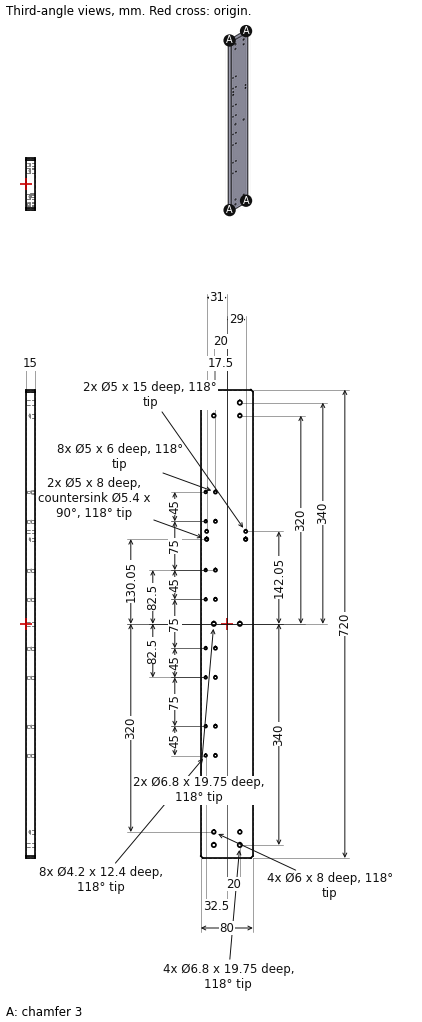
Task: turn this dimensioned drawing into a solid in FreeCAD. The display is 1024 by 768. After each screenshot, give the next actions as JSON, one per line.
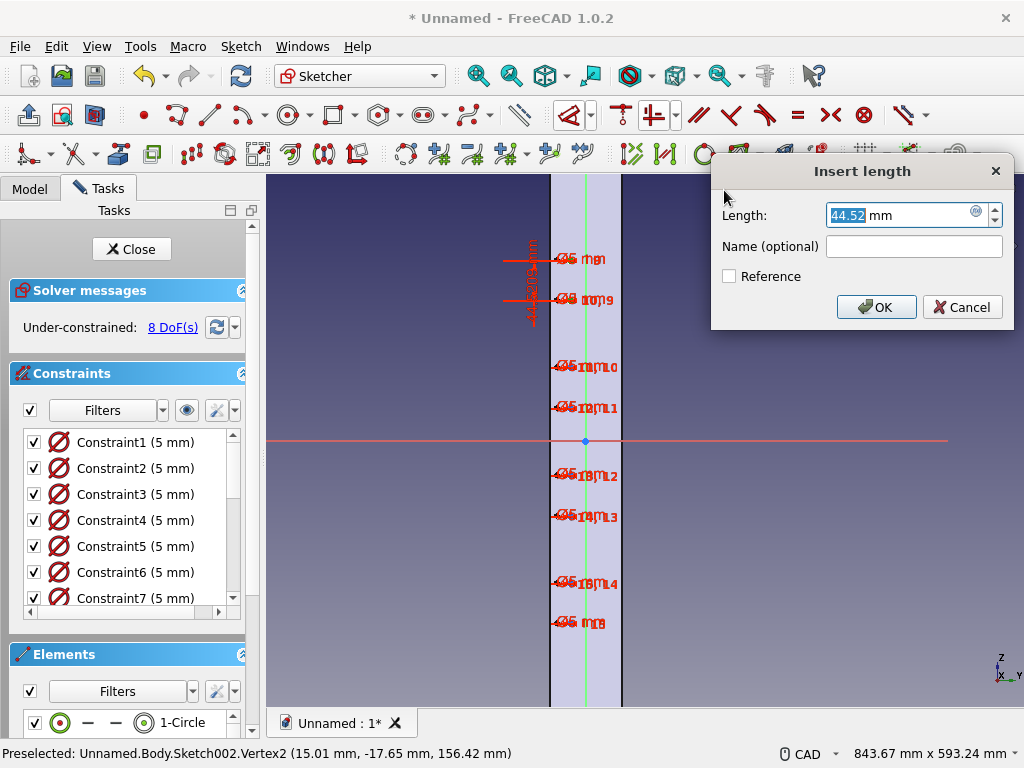
{"action": "type", "text": "45"}
{"action": "key", "text": "Return"}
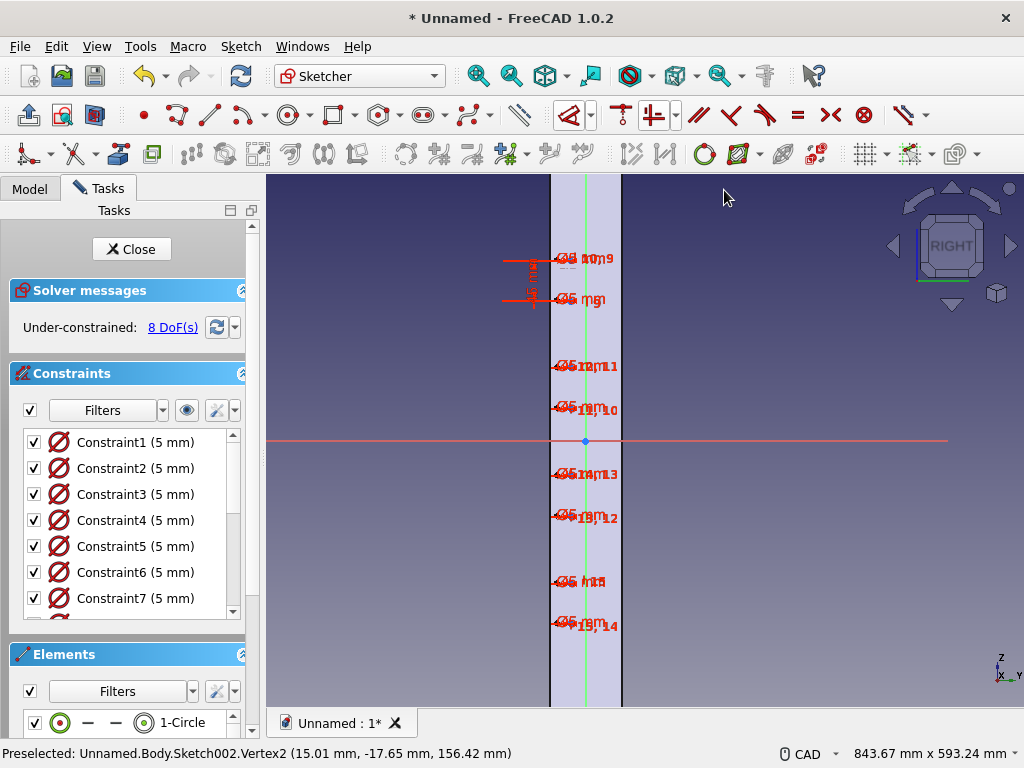
{"action": "left_click", "coordinate": [570, 301]}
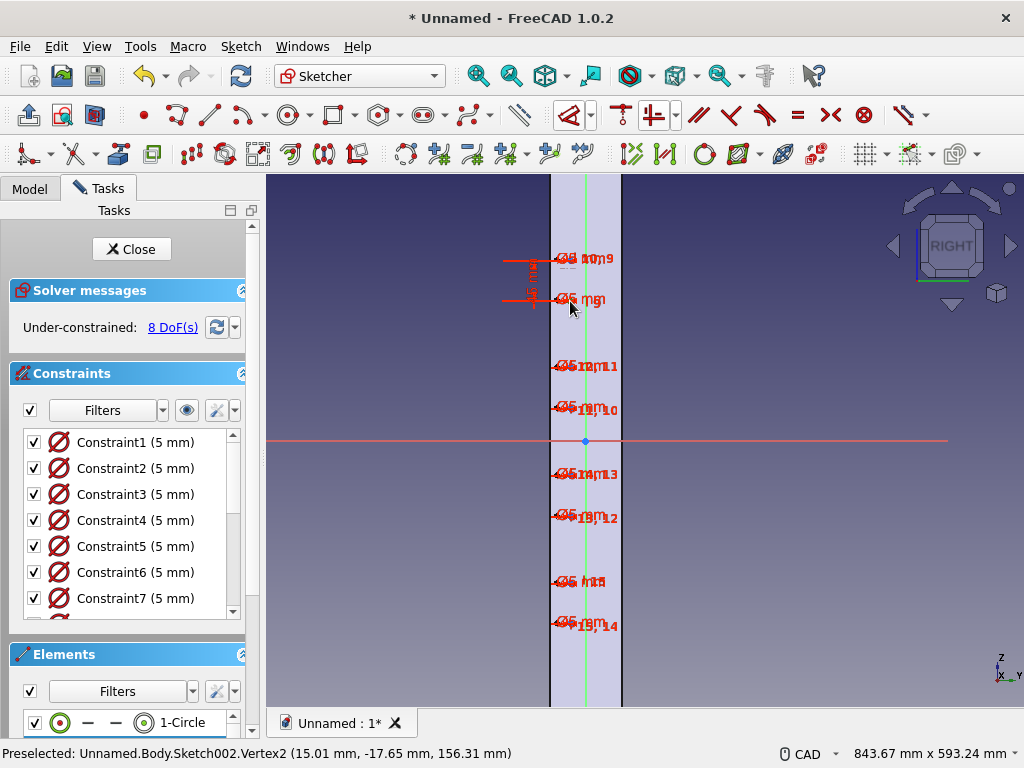
{"action": "left_click", "coordinate": [570, 368]}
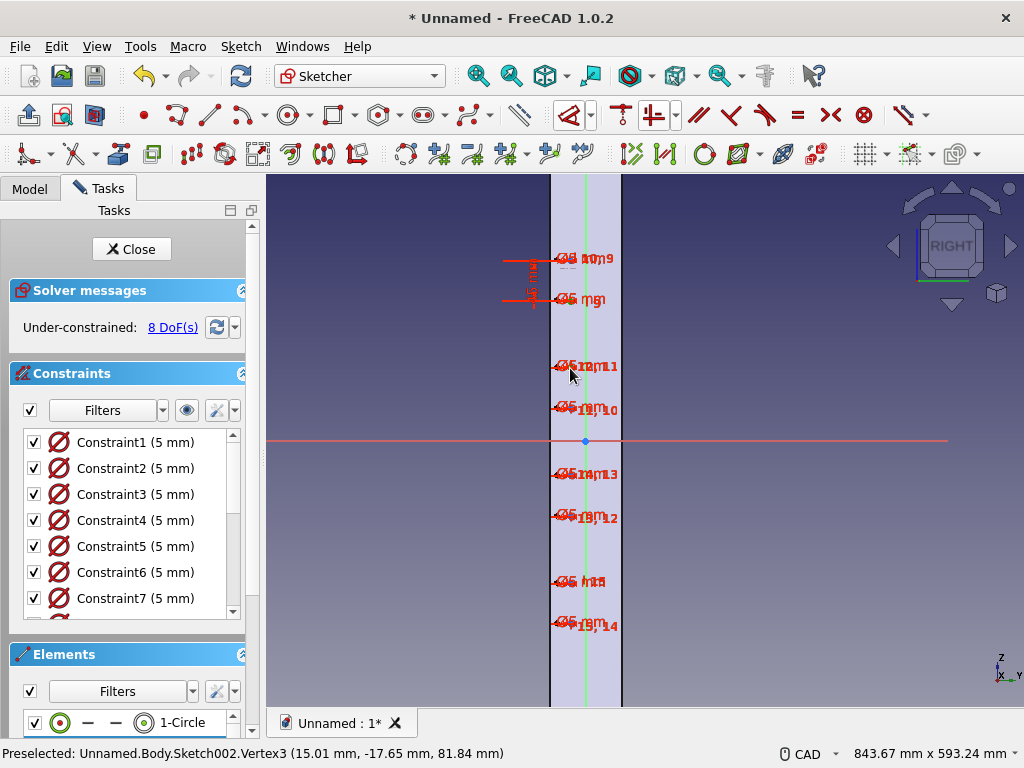
{"action": "left_click", "coordinate": [590, 116]}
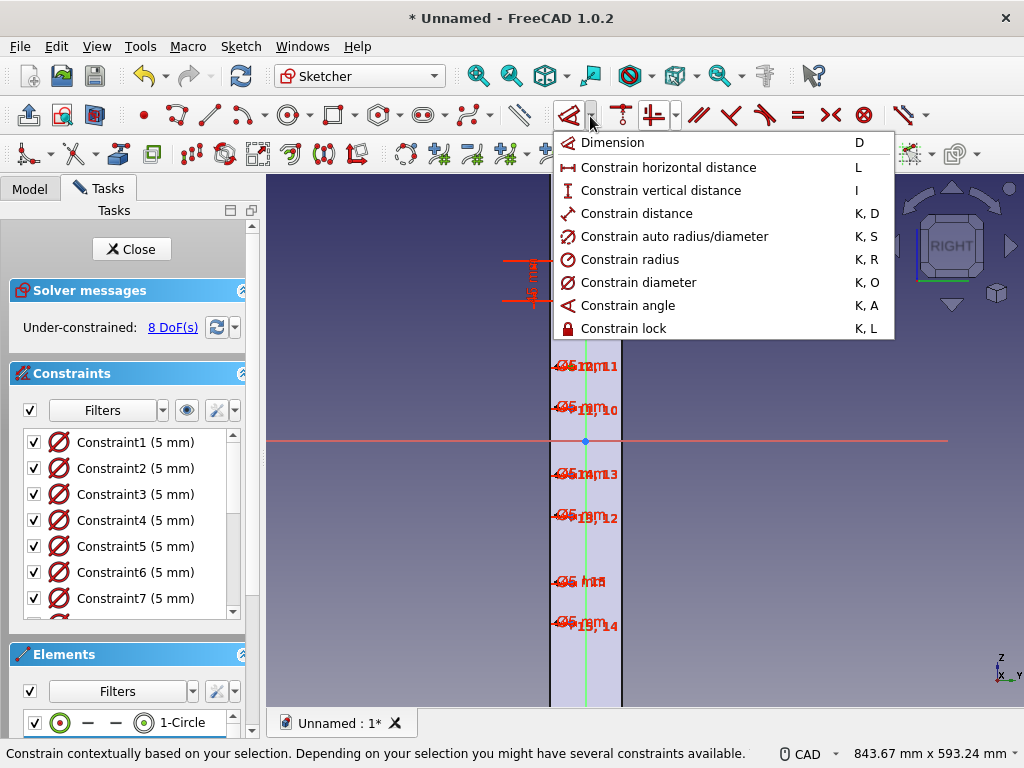
{"action": "left_click", "coordinate": [724, 190]}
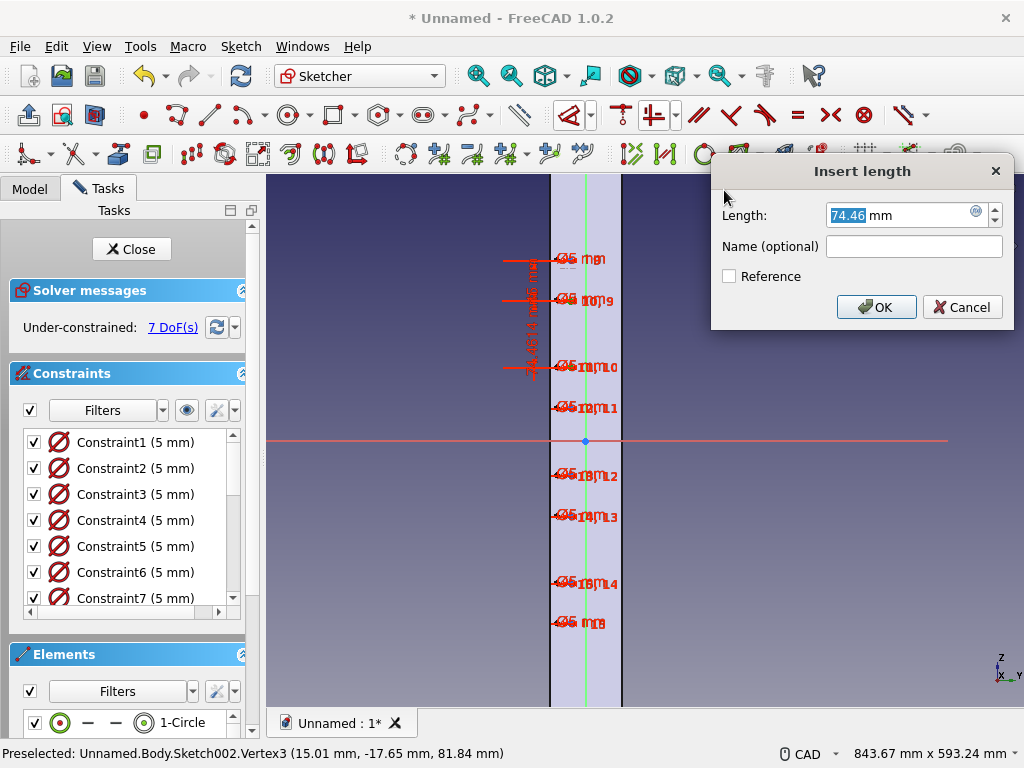
{"action": "type", "text": "75"}
{"action": "key", "text": "Return"}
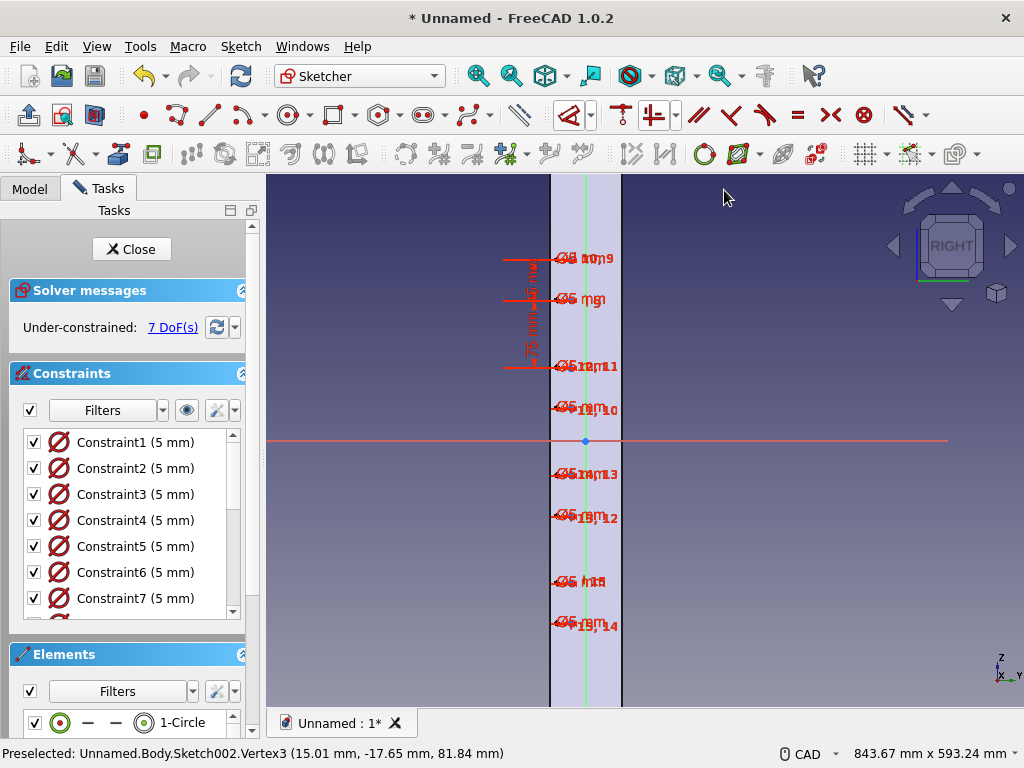
{"action": "left_click", "coordinate": [570, 368]}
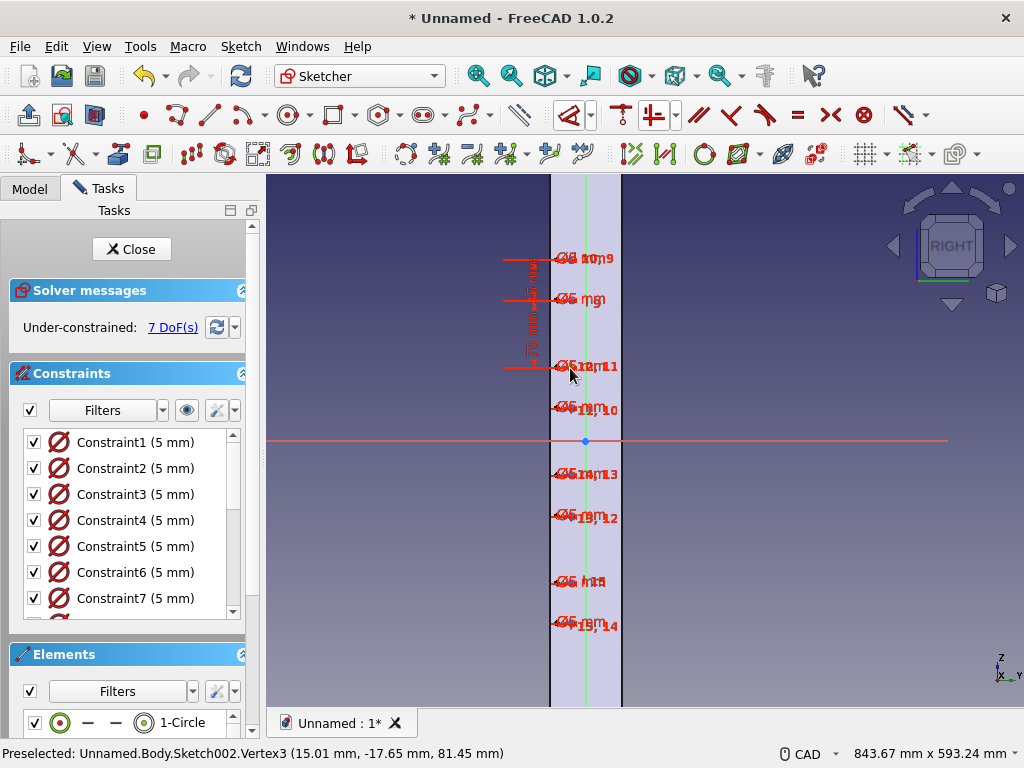
{"action": "left_click", "coordinate": [570, 409]}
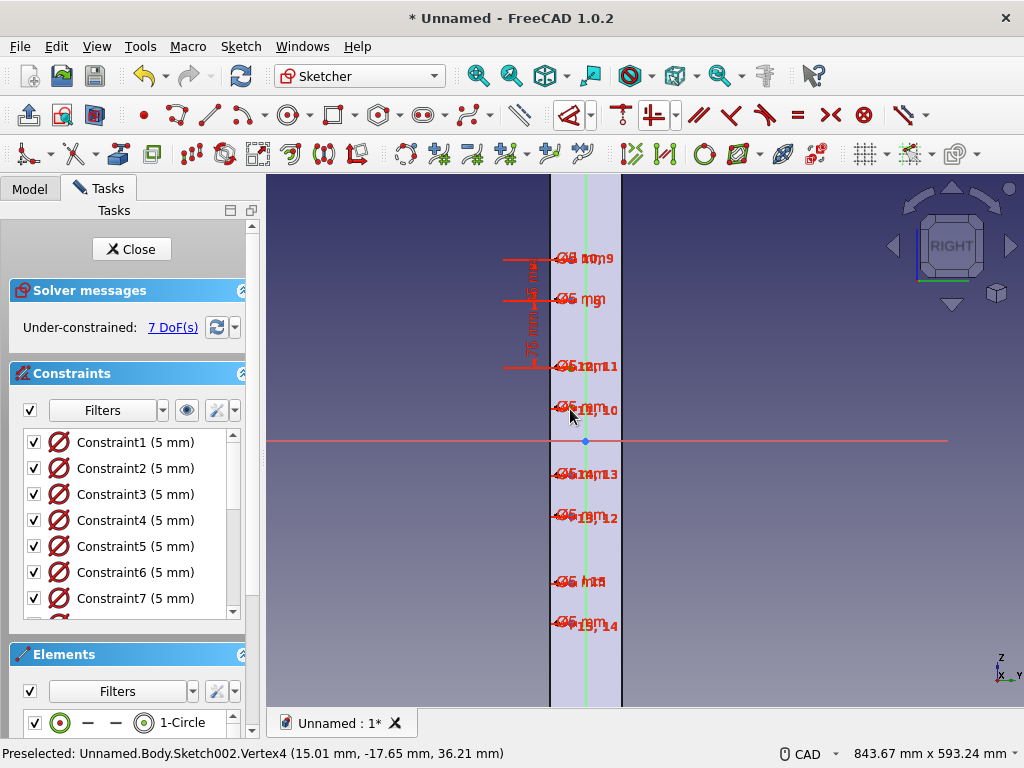
{"action": "left_click", "coordinate": [590, 116]}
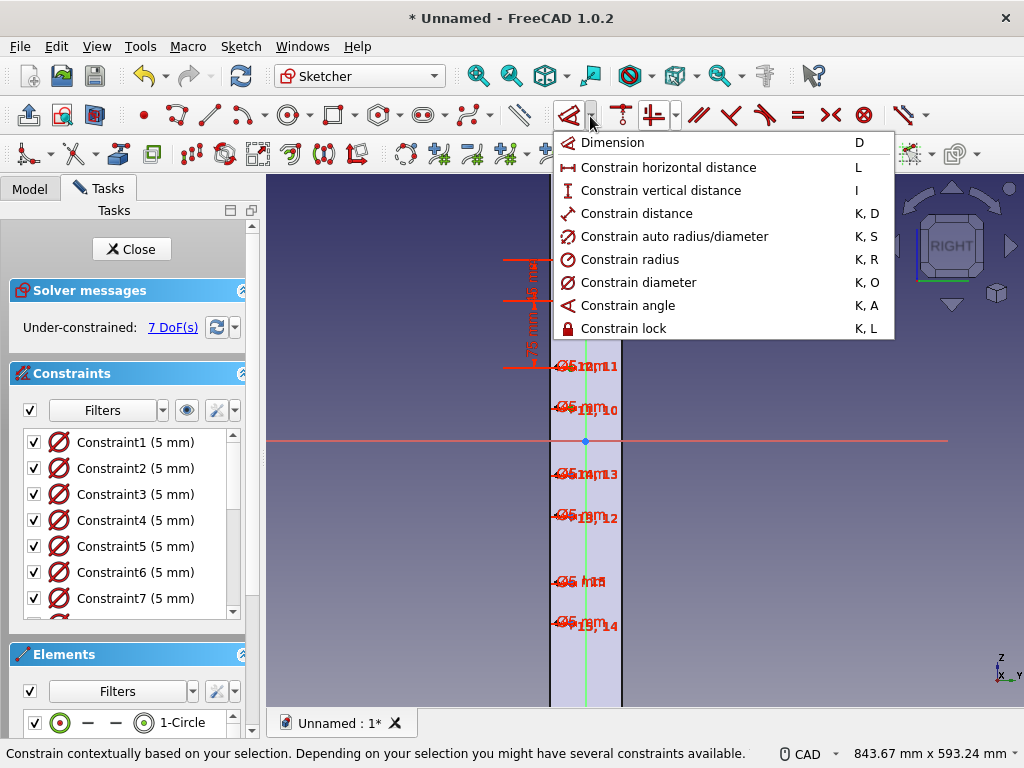
{"action": "left_click", "coordinate": [724, 190]}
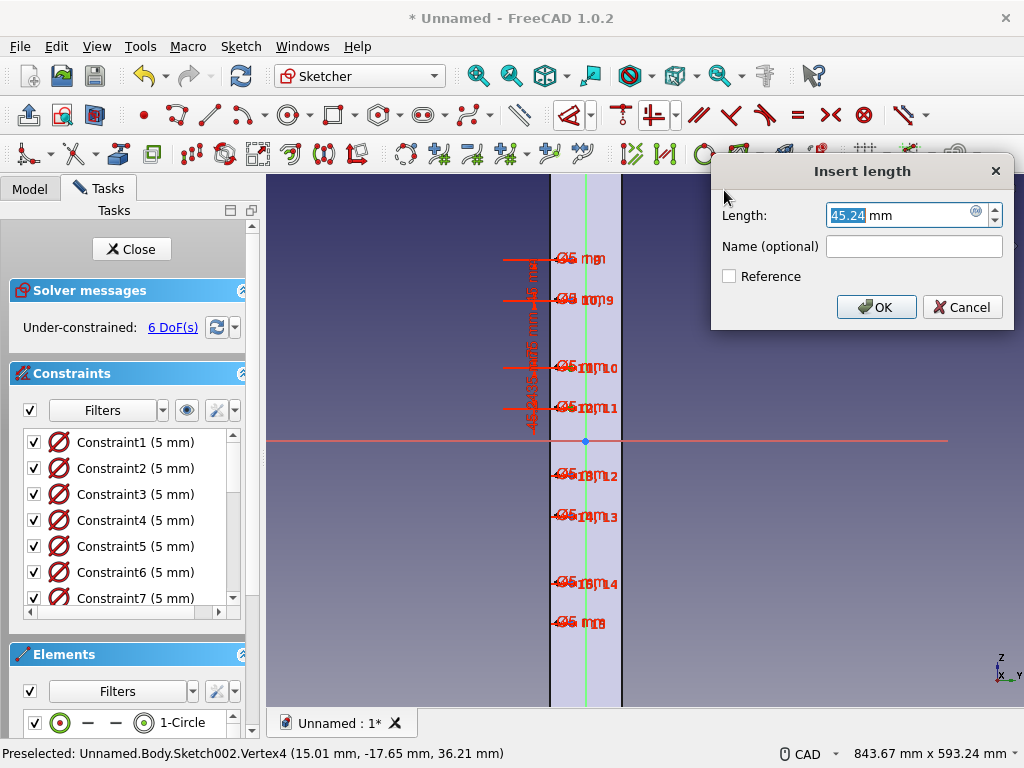
{"action": "type", "text": "45"}
{"action": "key", "text": "Return"}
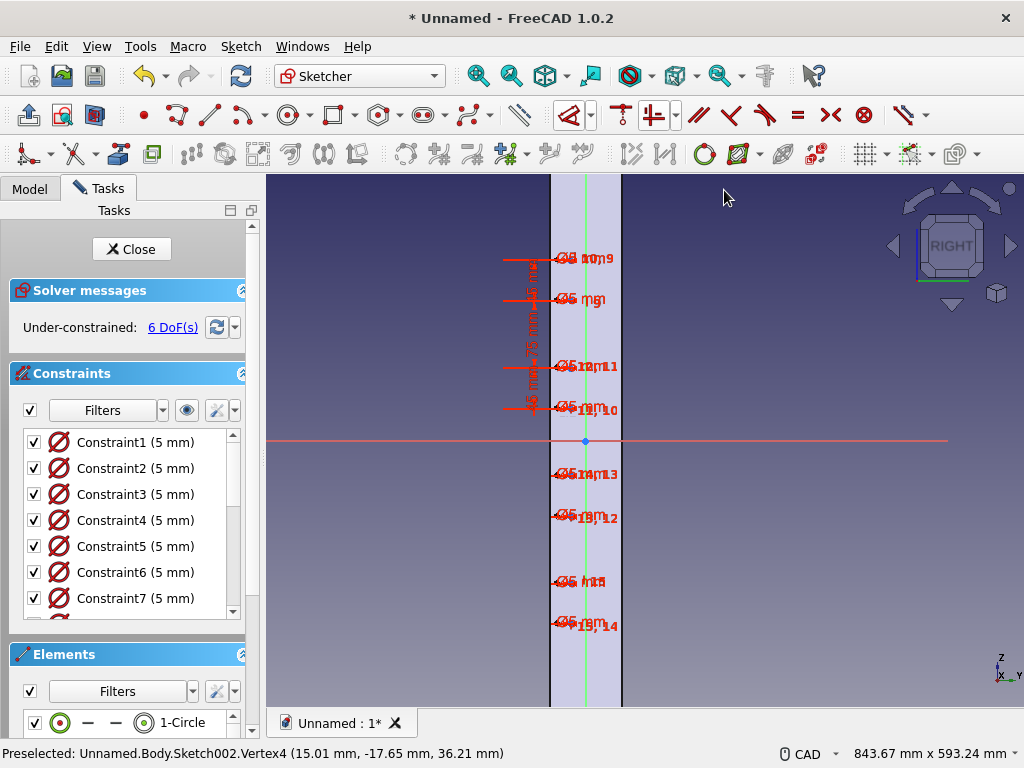
{"action": "left_click", "coordinate": [570, 409]}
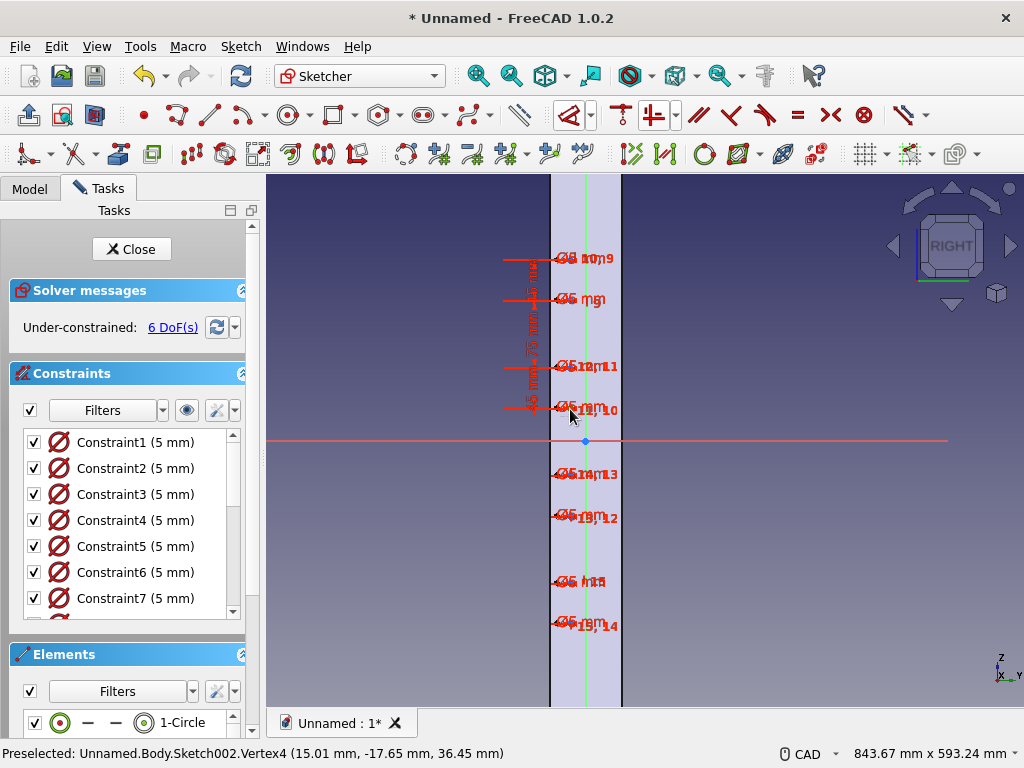
{"action": "left_click", "coordinate": [570, 476]}